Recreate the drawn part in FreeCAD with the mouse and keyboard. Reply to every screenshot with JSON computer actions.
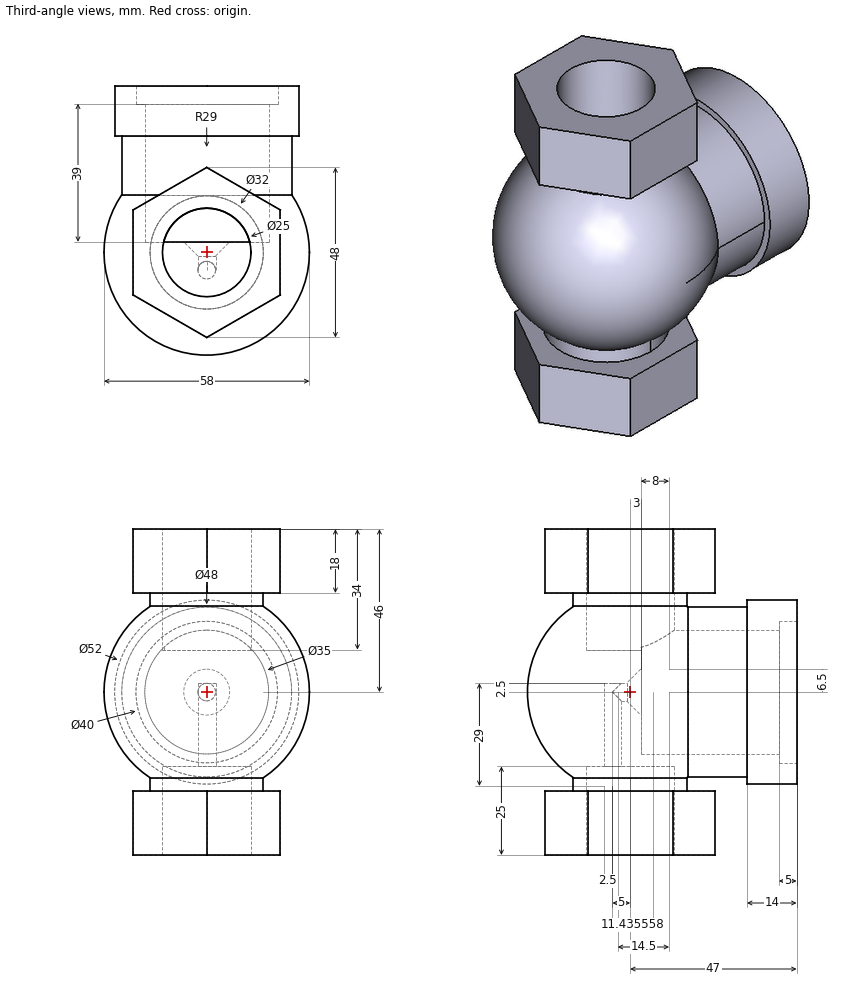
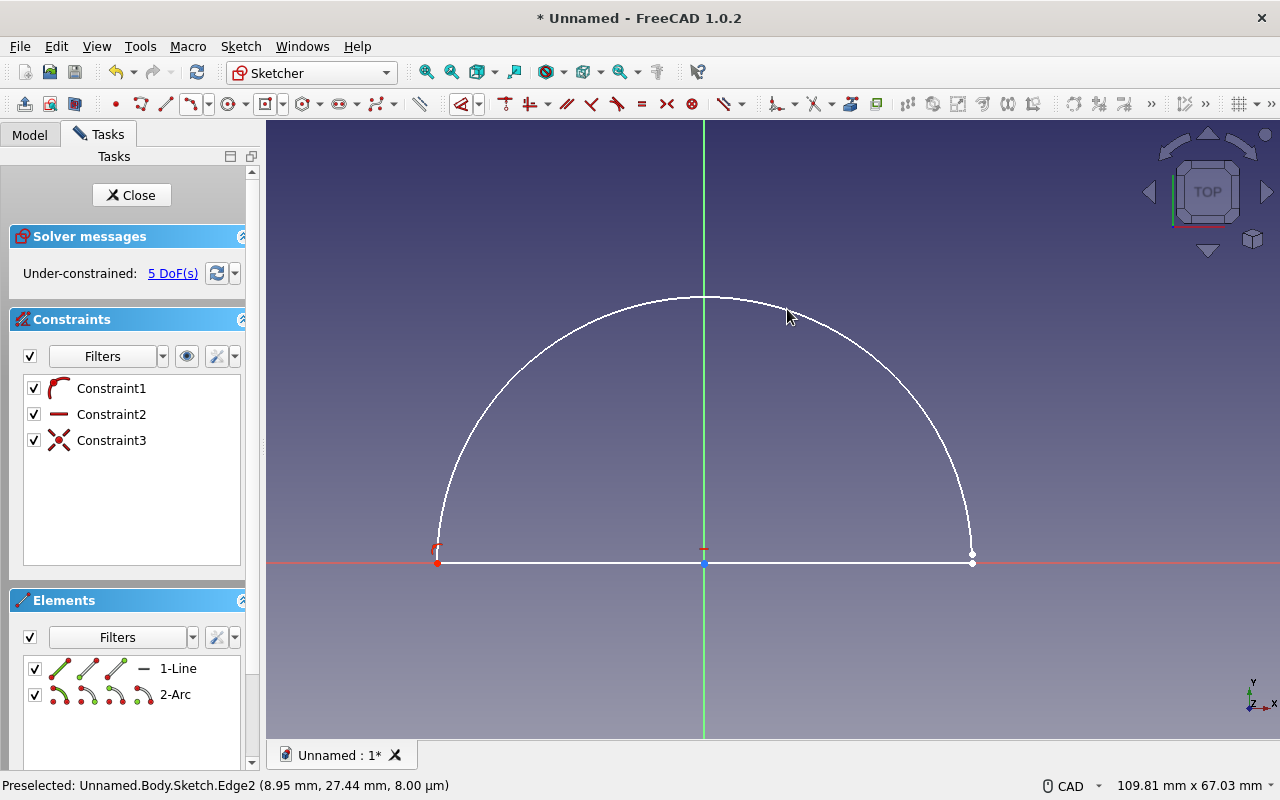
{"action": "left_click_drag", "start_coordinate": [694, 553], "coordinate": [715, 575]}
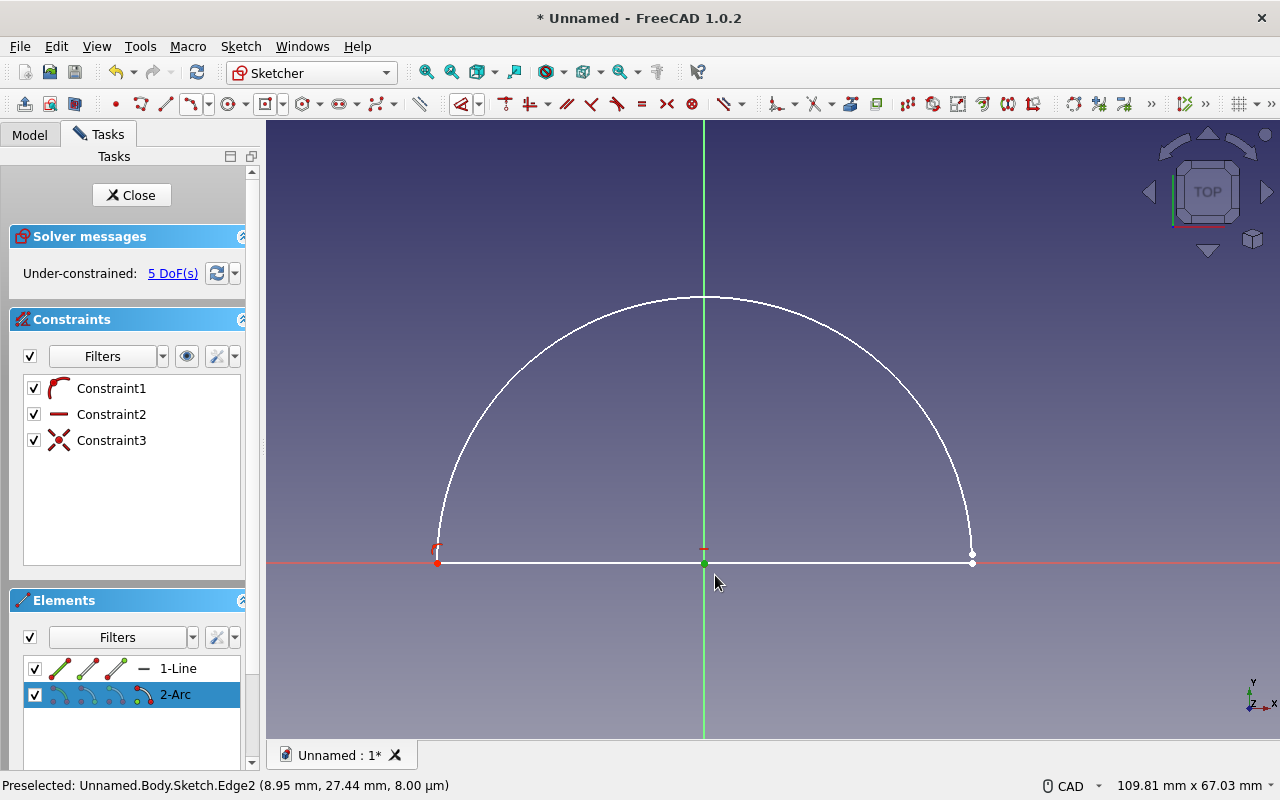
{"action": "left_click", "coordinate": [505, 104]}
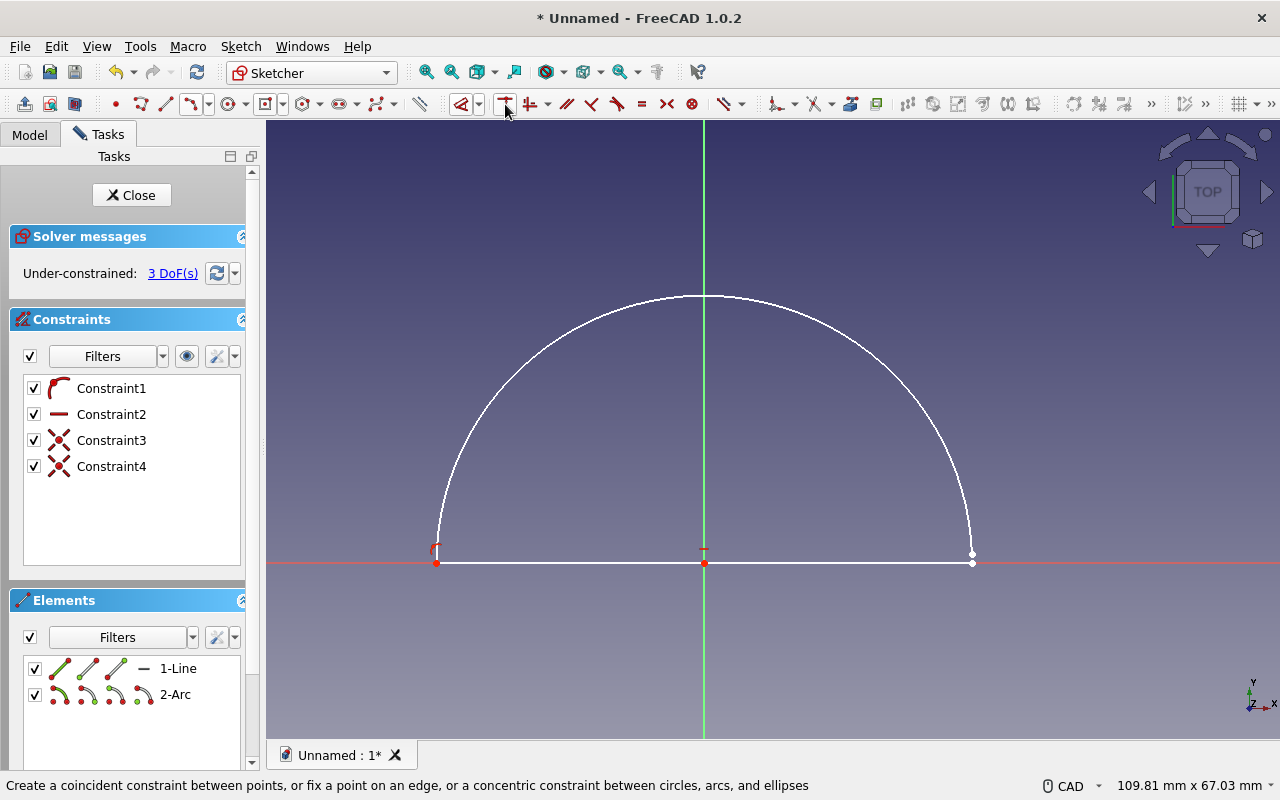
{"action": "left_click", "coordinate": [857, 343]}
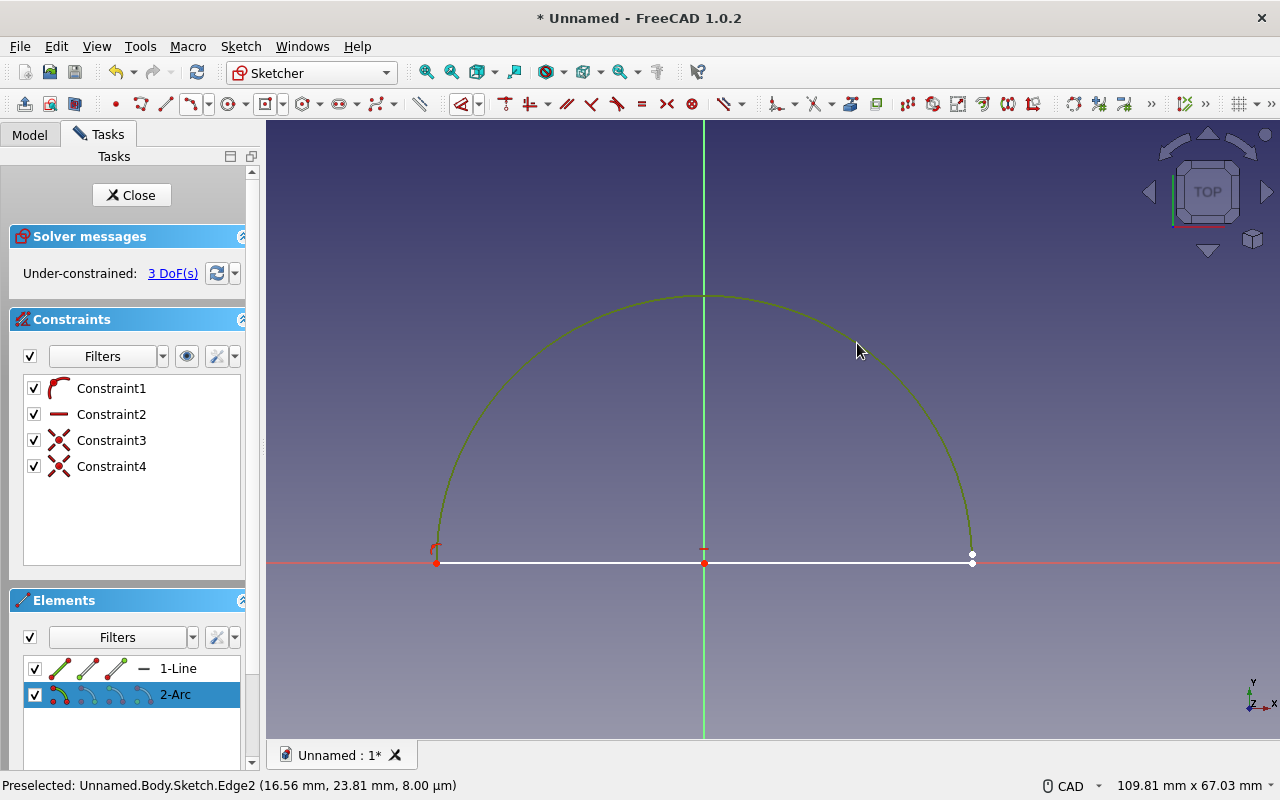
{"action": "left_click", "coordinate": [478, 104]}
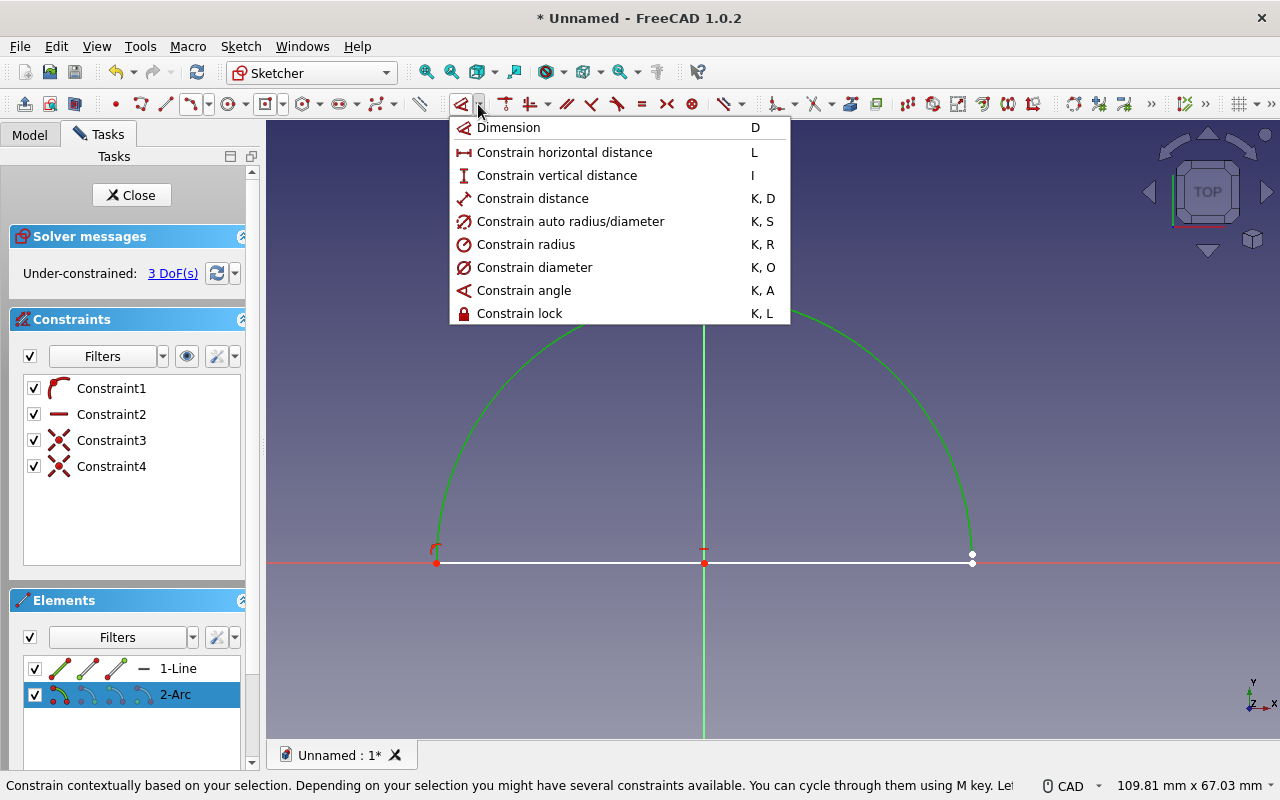
{"action": "left_click", "coordinate": [620, 244]}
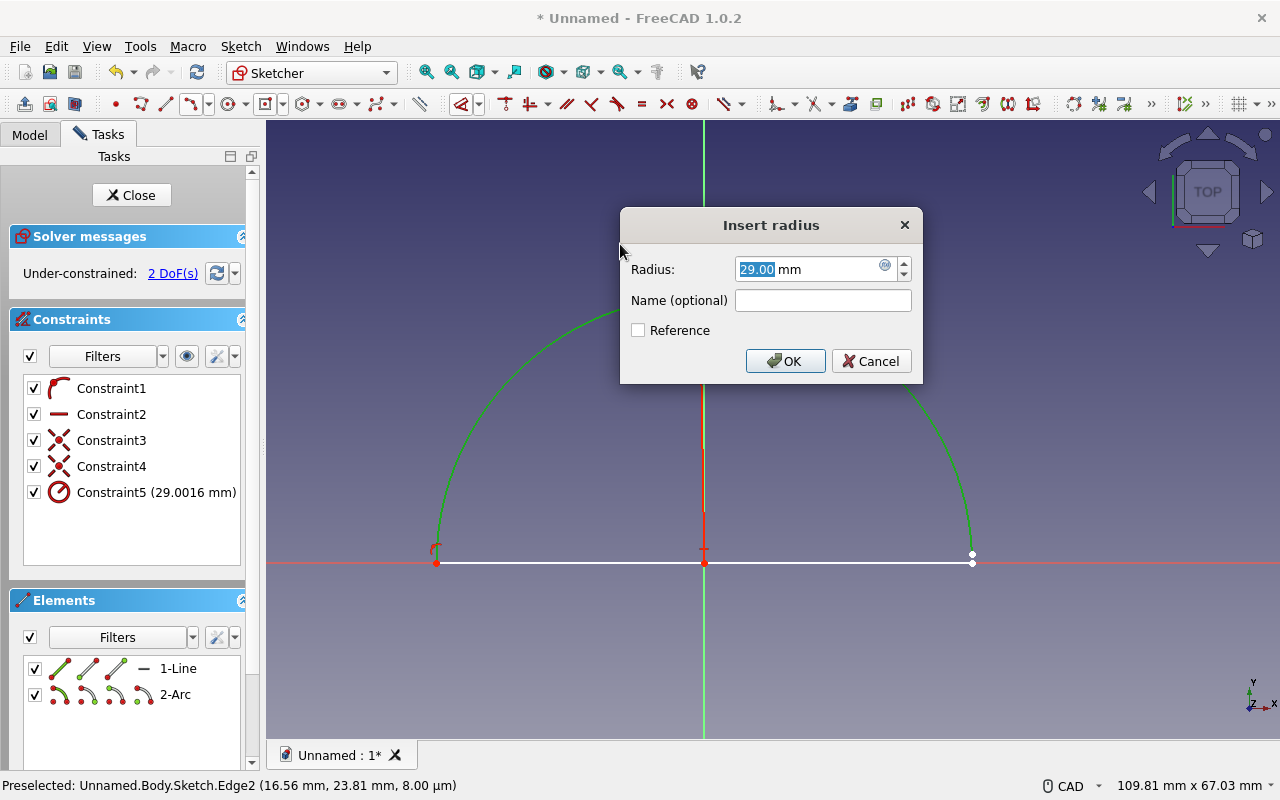
{"action": "type", "text": "29"}
{"action": "key", "text": "Return"}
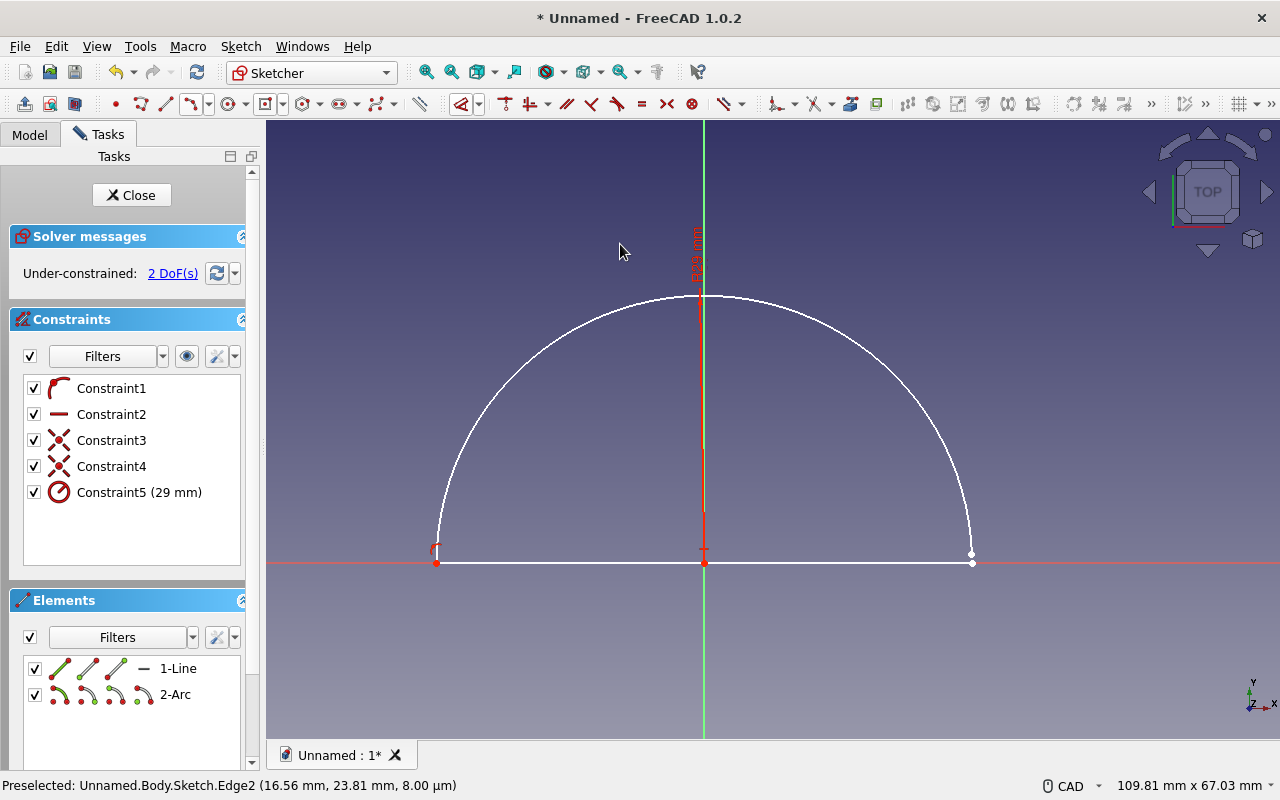
{"action": "left_click", "coordinate": [972, 555]}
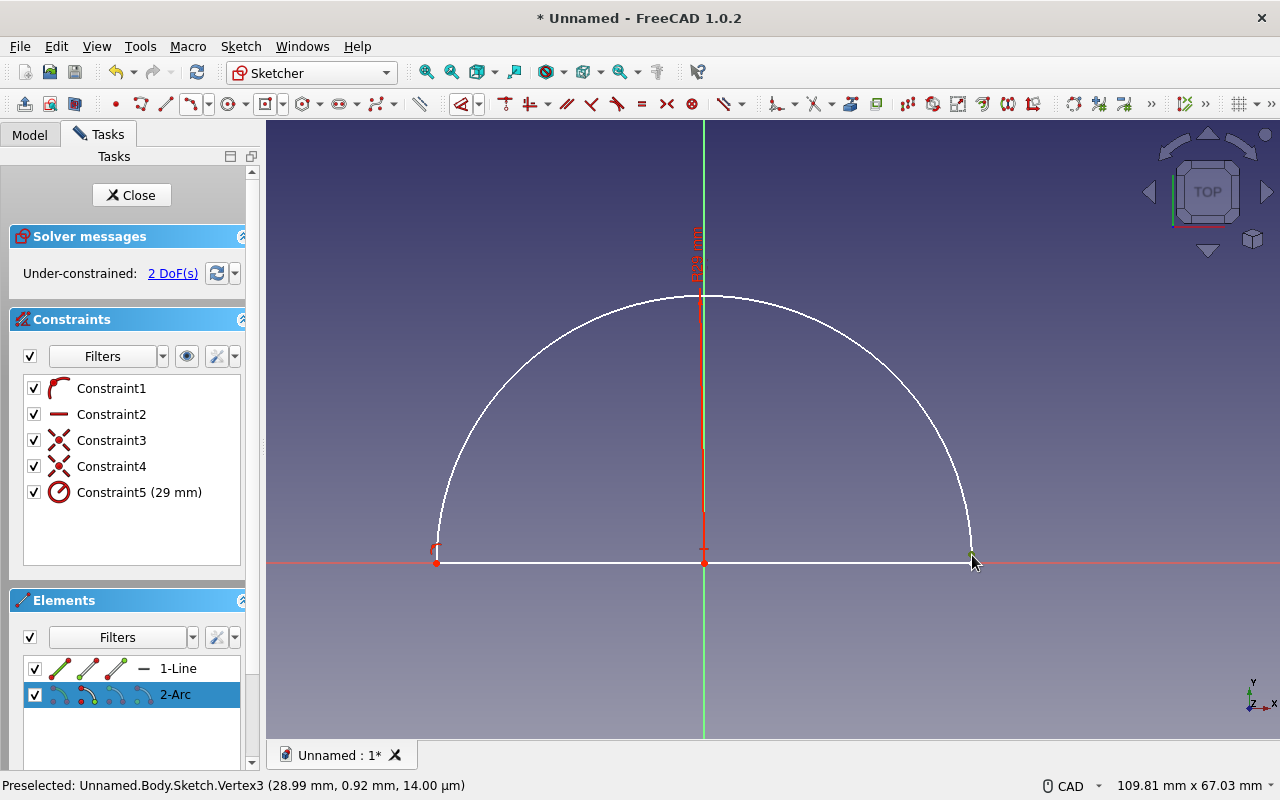
{"action": "left_click", "coordinate": [353, 563]}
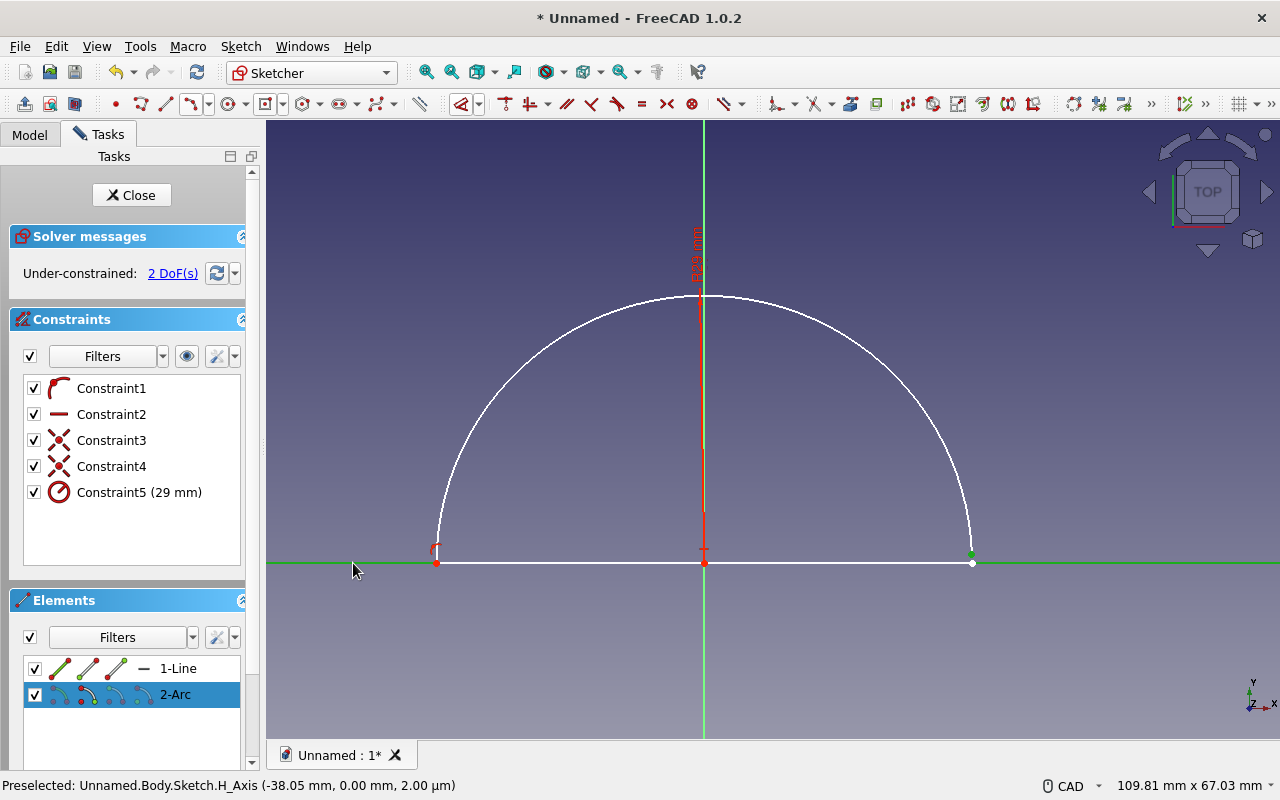
{"action": "left_click", "coordinate": [505, 104]}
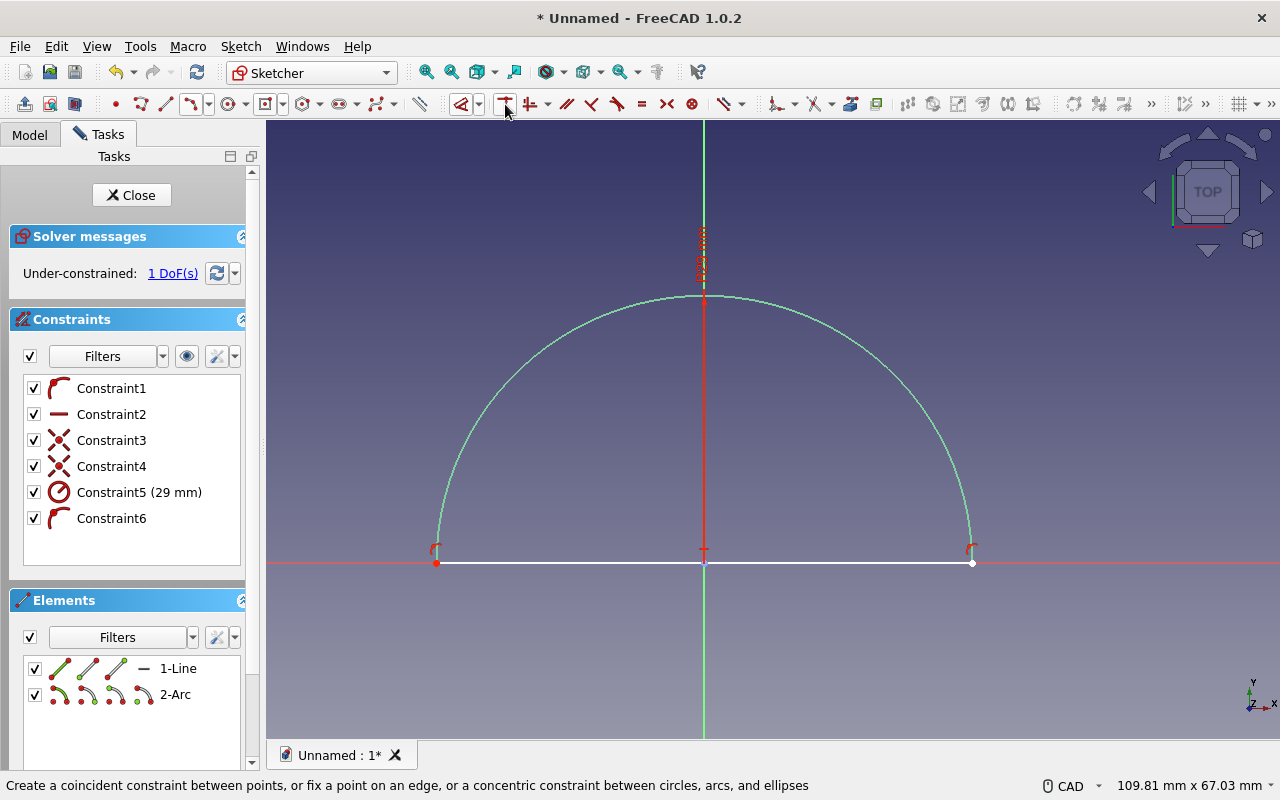
{"action": "left_click", "coordinate": [597, 563]}